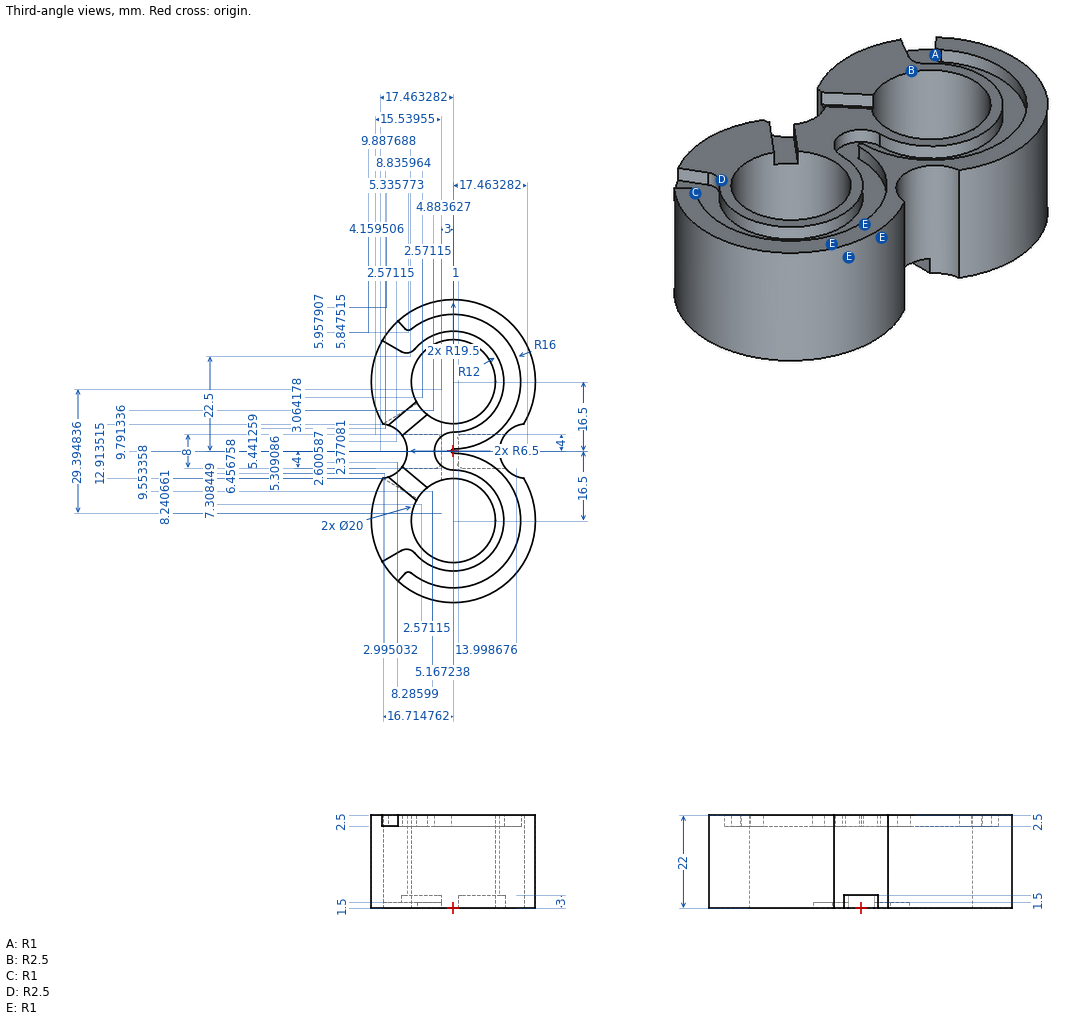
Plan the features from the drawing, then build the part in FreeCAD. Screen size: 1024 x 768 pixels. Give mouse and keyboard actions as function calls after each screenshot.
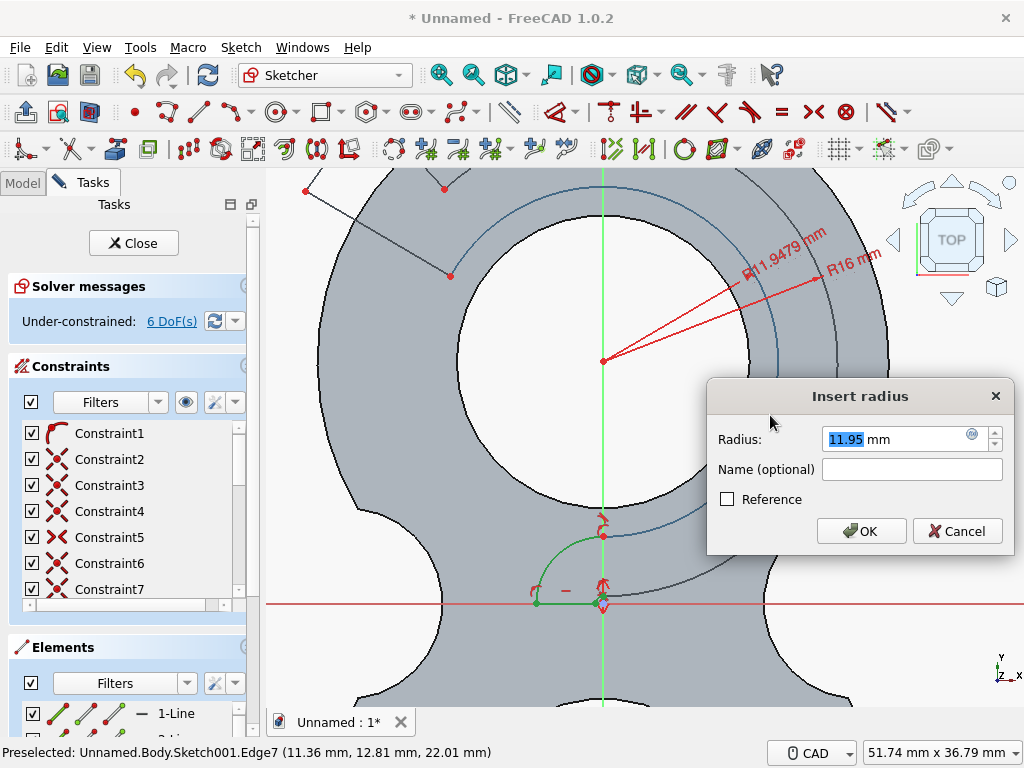
text(12)
key(Return)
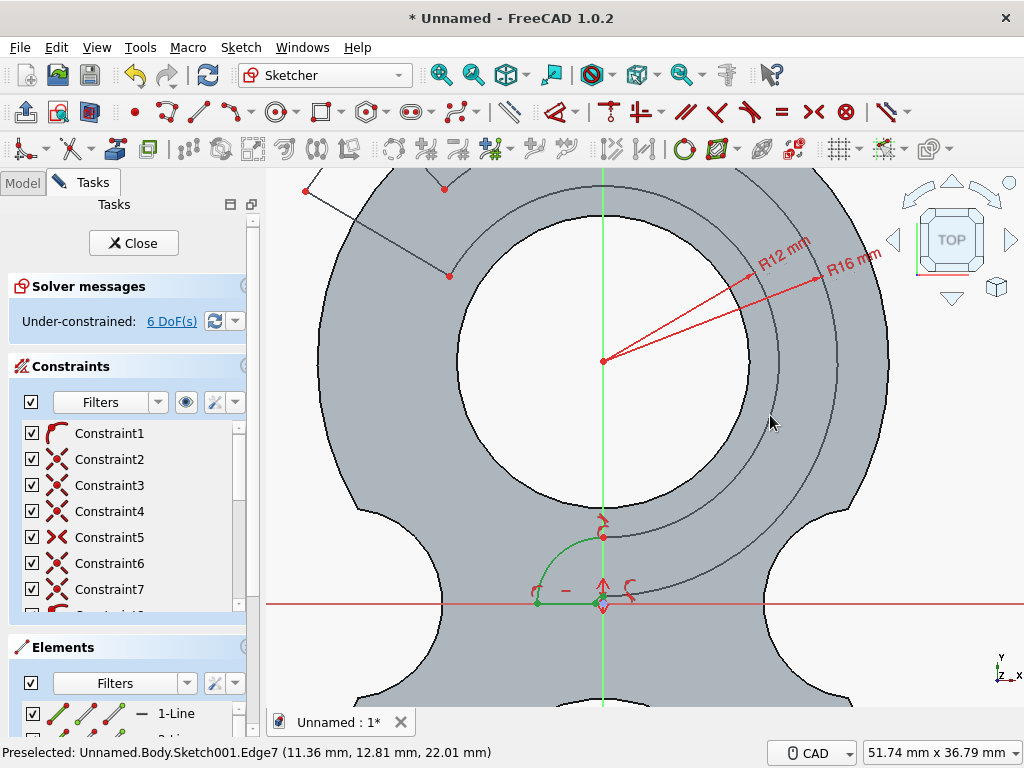
click(450, 276)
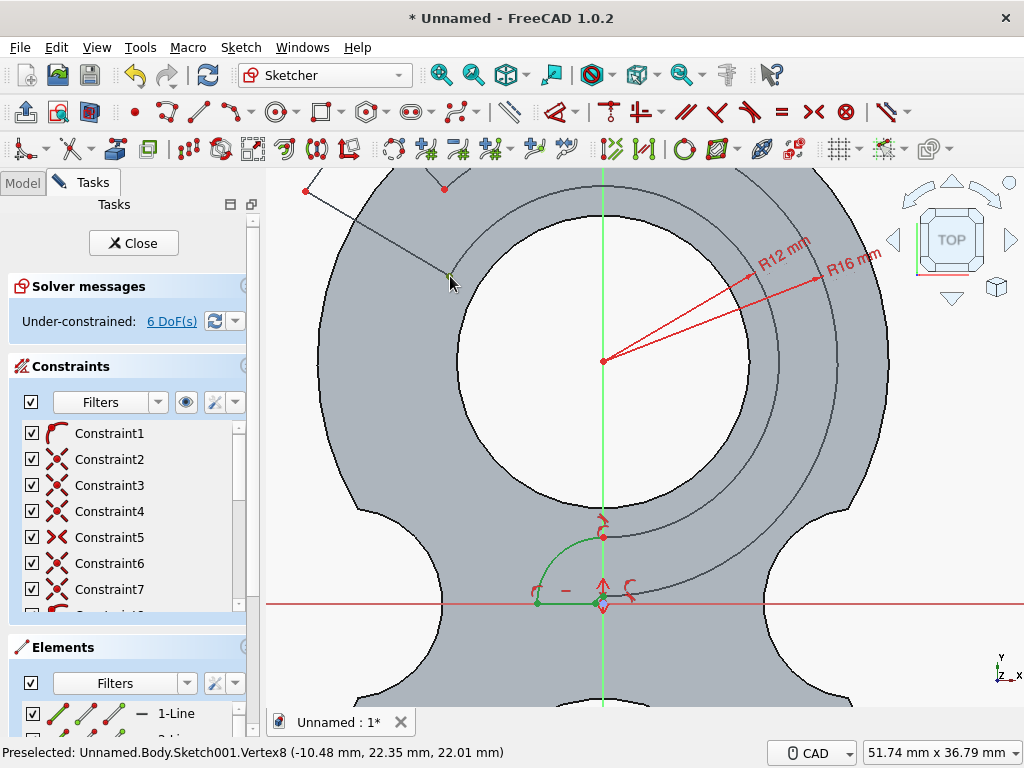
key(i)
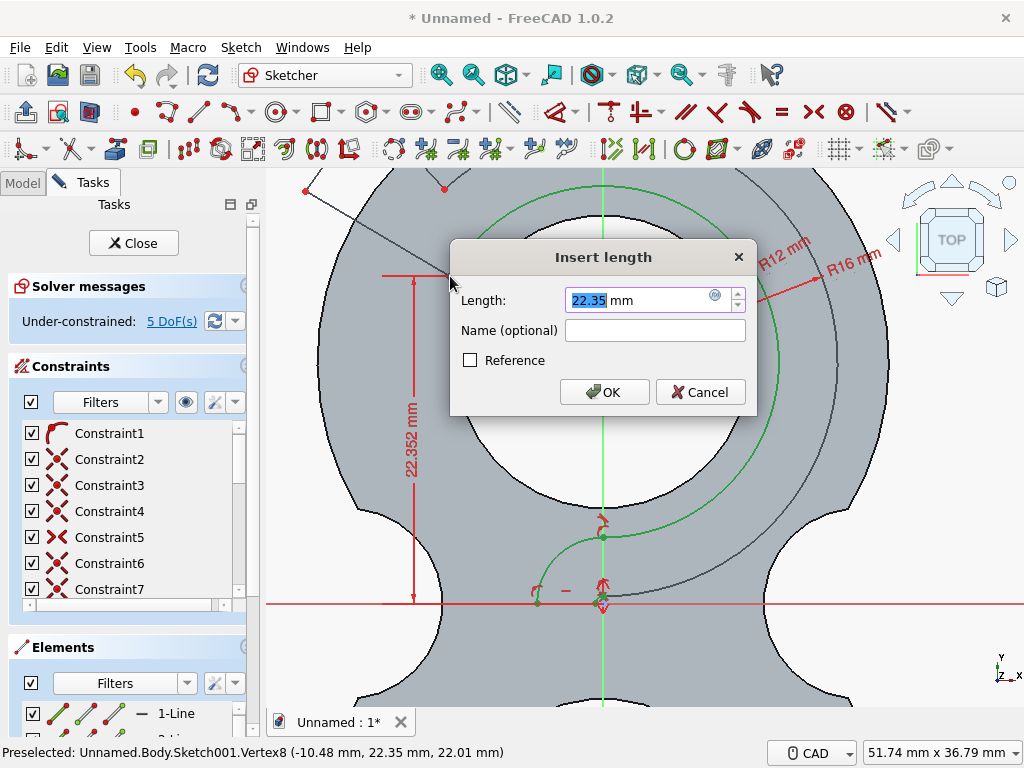
text(22.5)
key(Return)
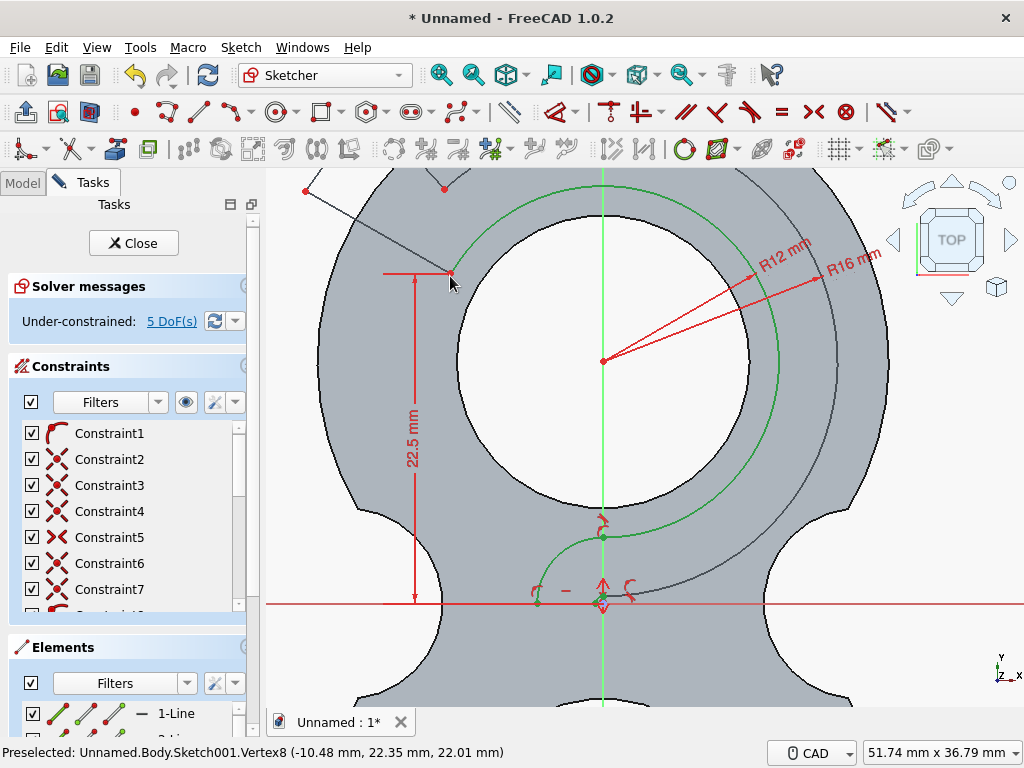
scroll(602, 609, down, 2)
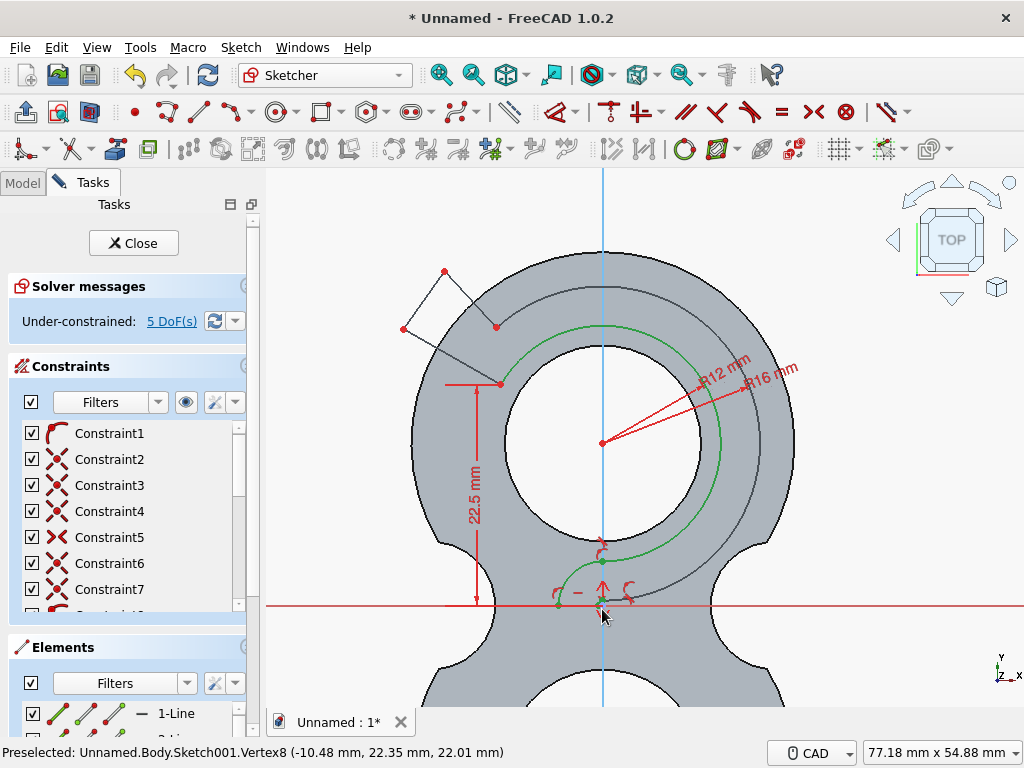
click(481, 311)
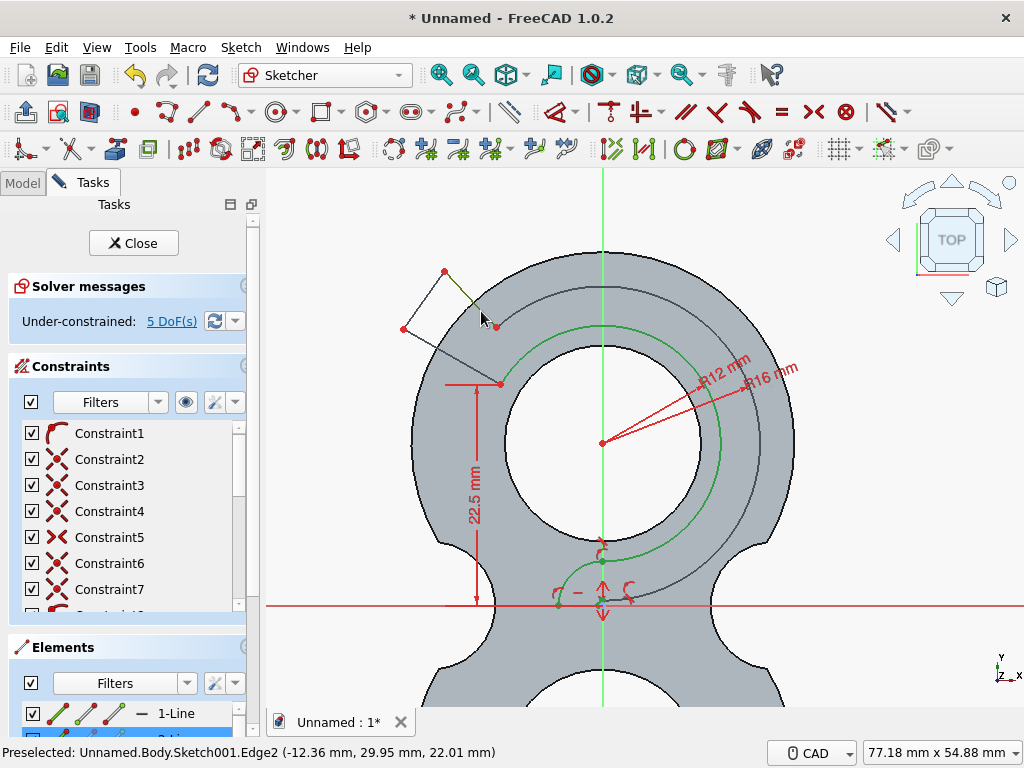
key(l)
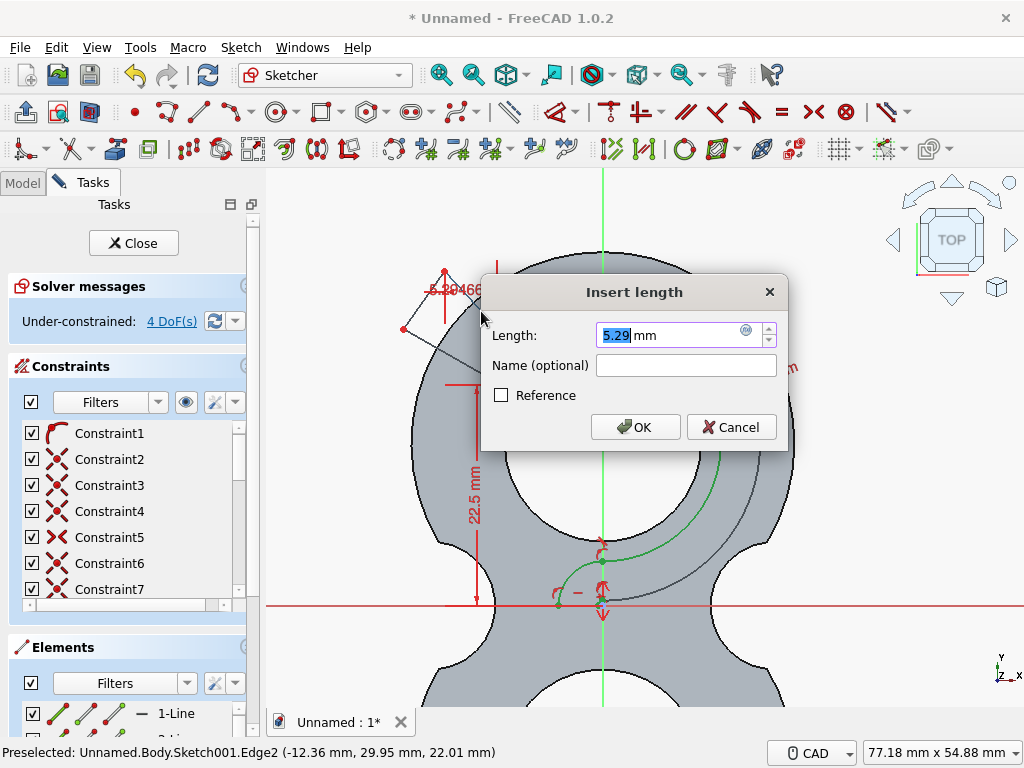
text(5.335773)
key(Return)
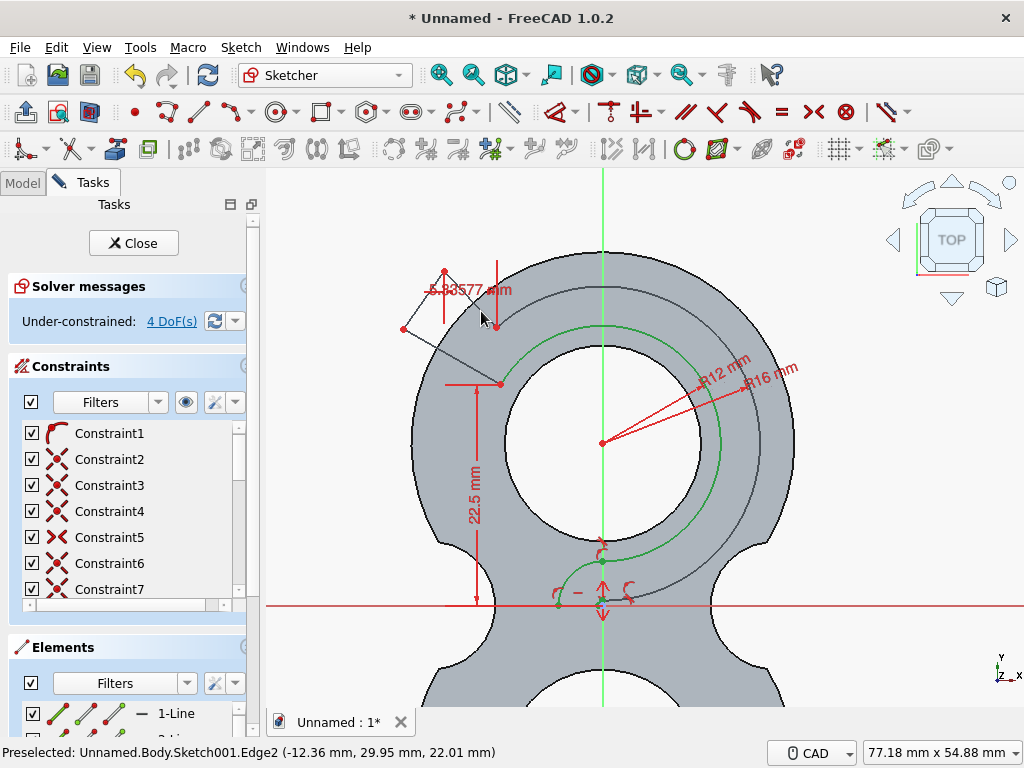
click(481, 311)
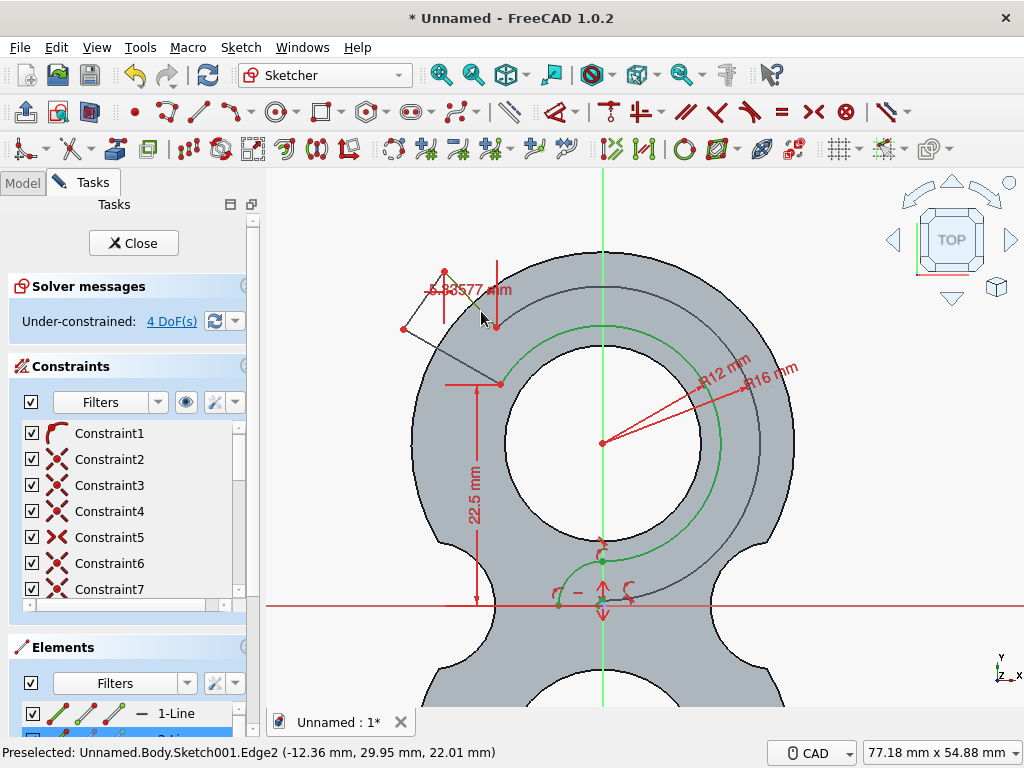
key(i)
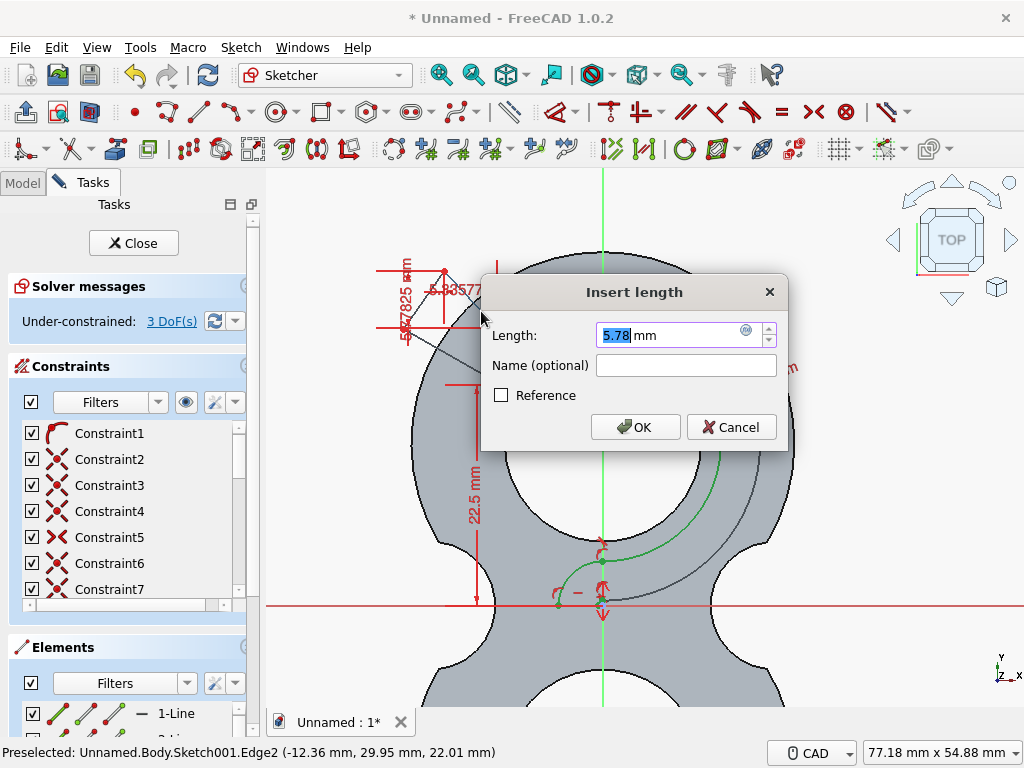
text(5.847515)
key(Return)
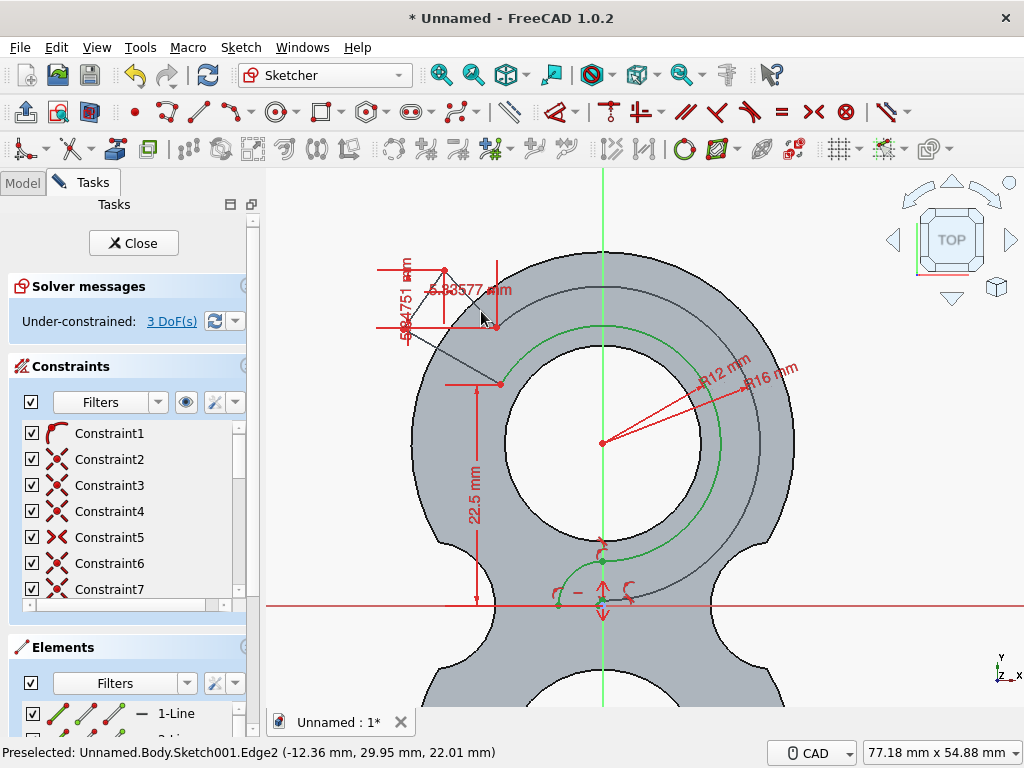
click(428, 294)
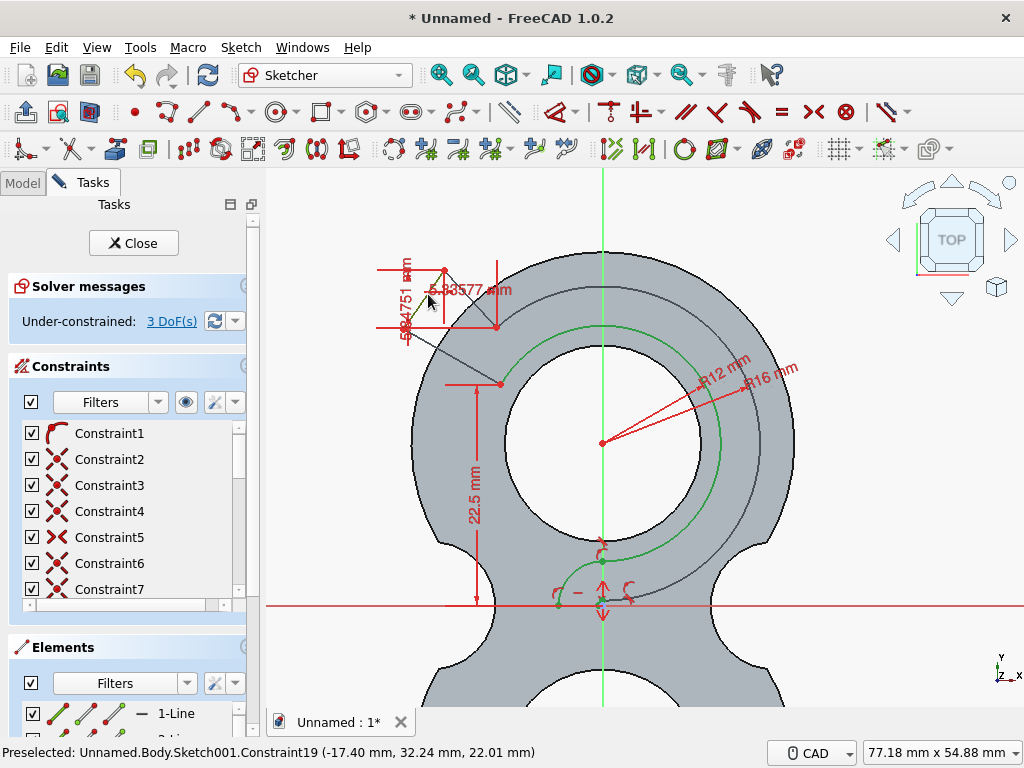
key(l)